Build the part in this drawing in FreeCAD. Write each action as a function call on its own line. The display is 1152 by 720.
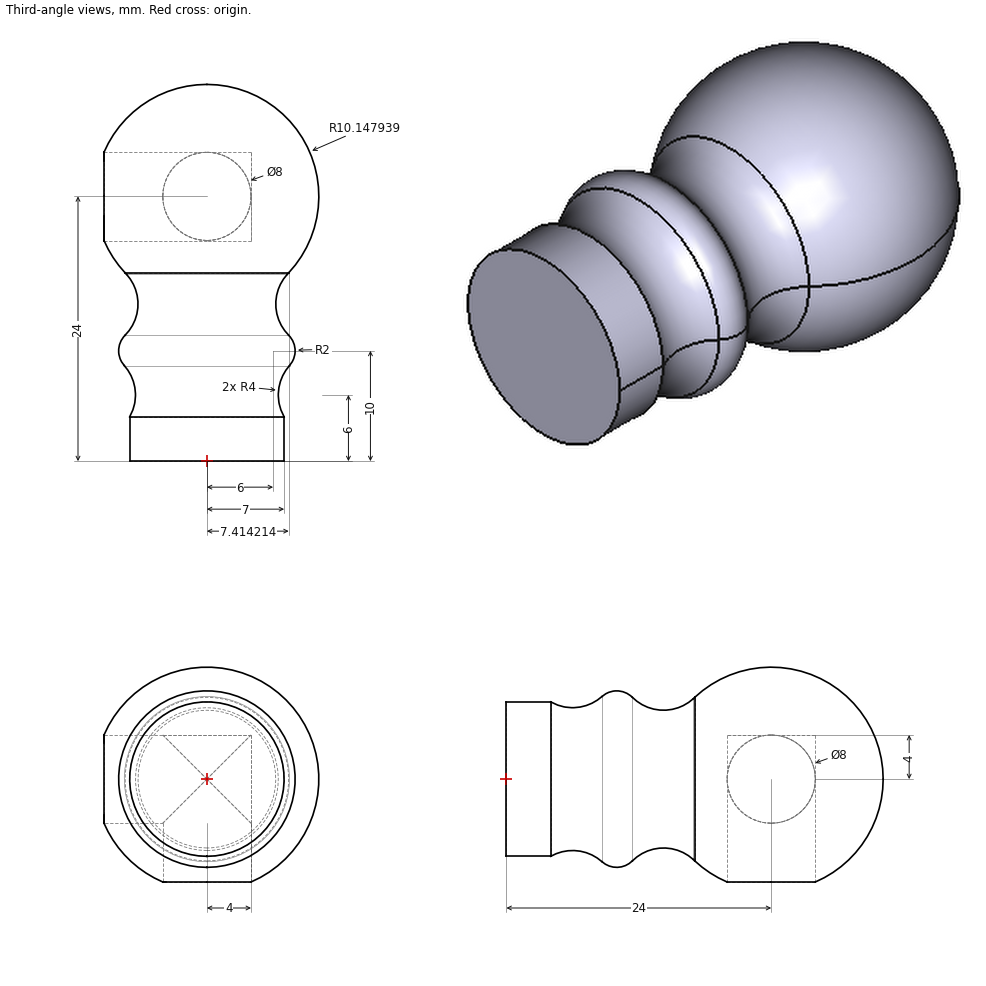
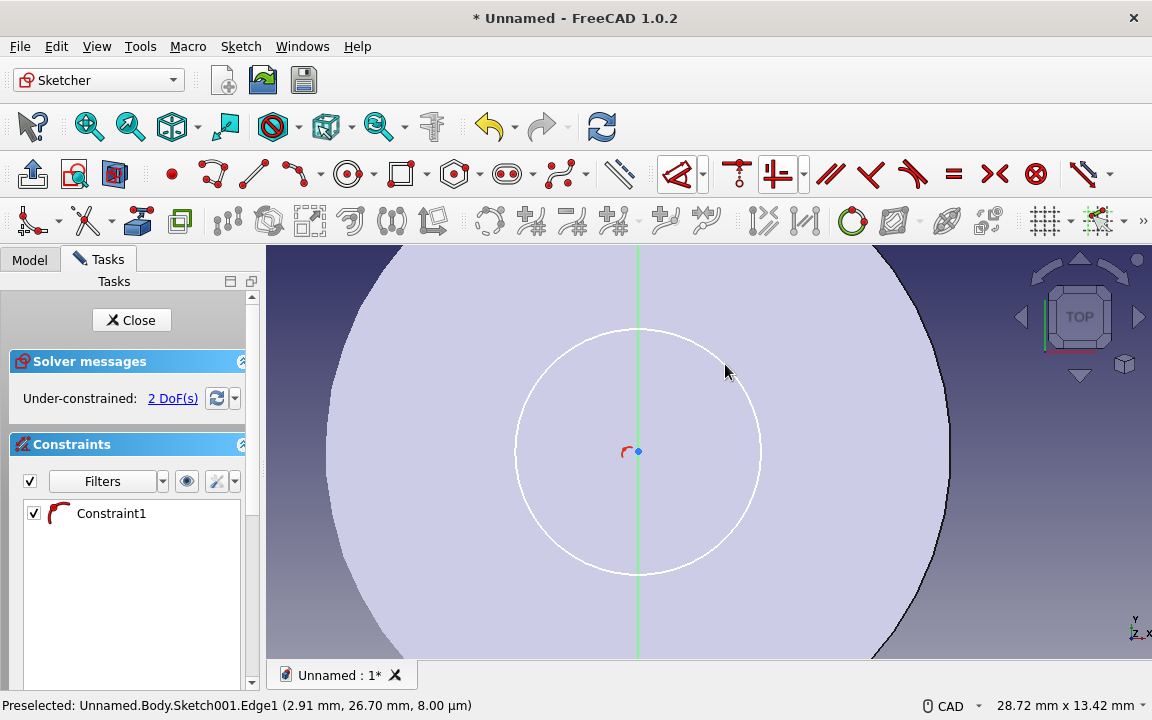
click(725, 365)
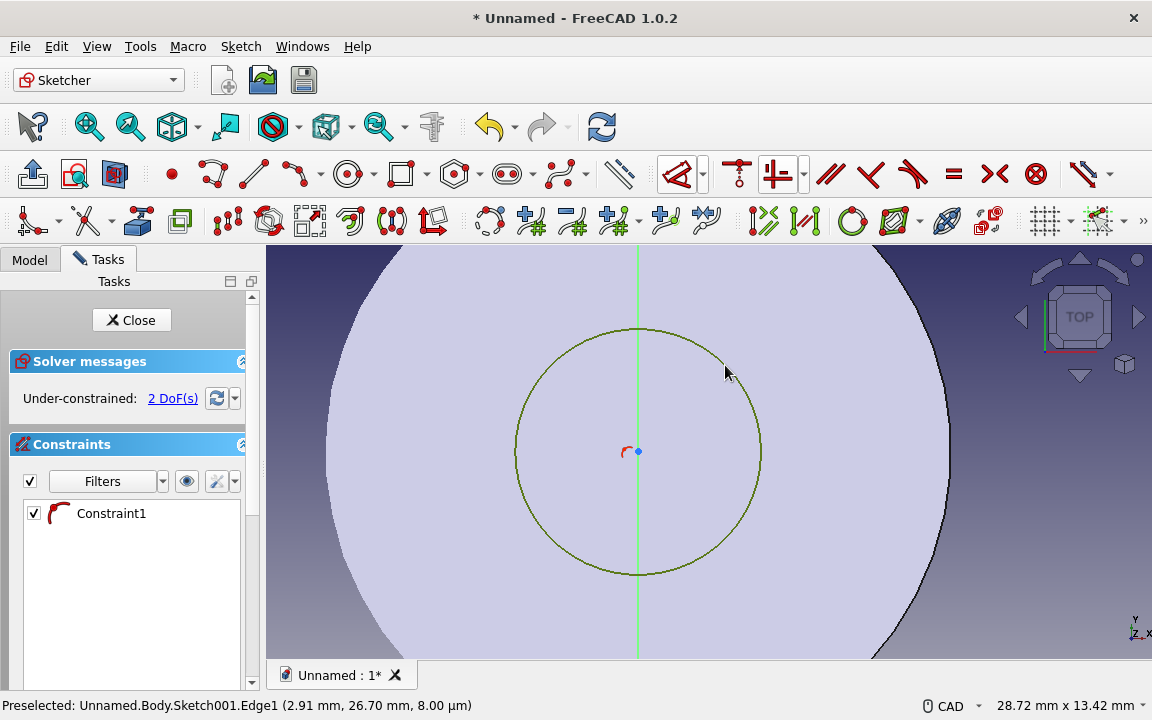
key(k)
key(o)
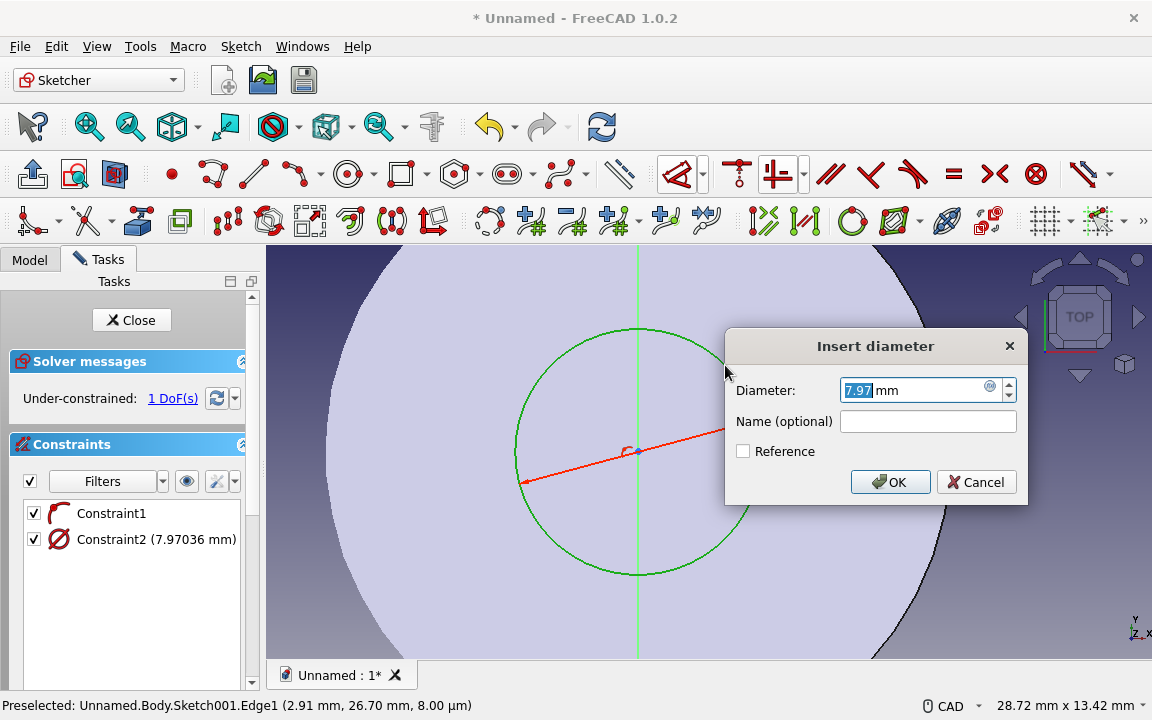
text(8)
key(Return)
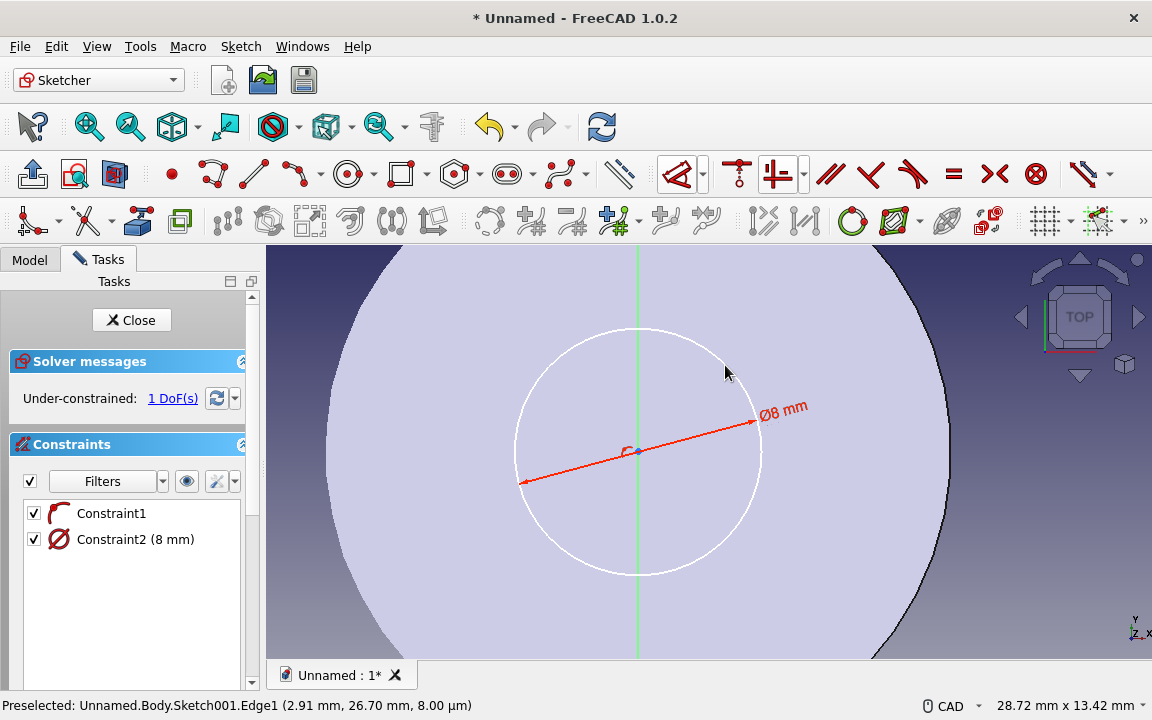
click(638, 452)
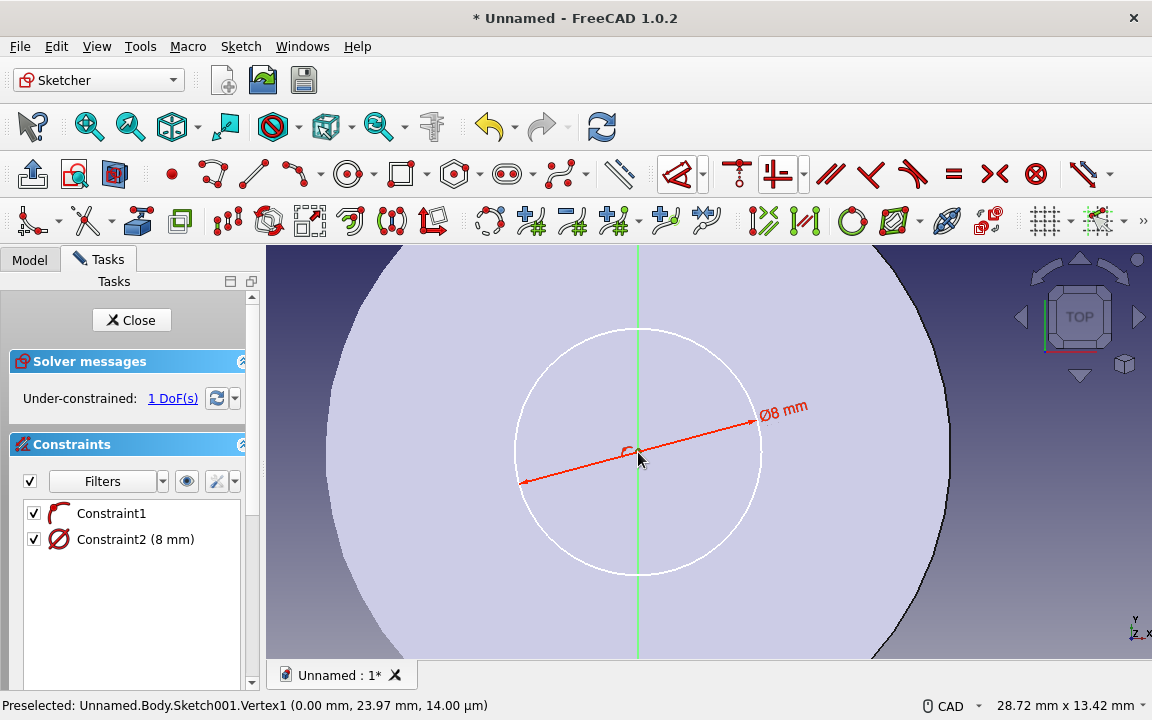
key(i)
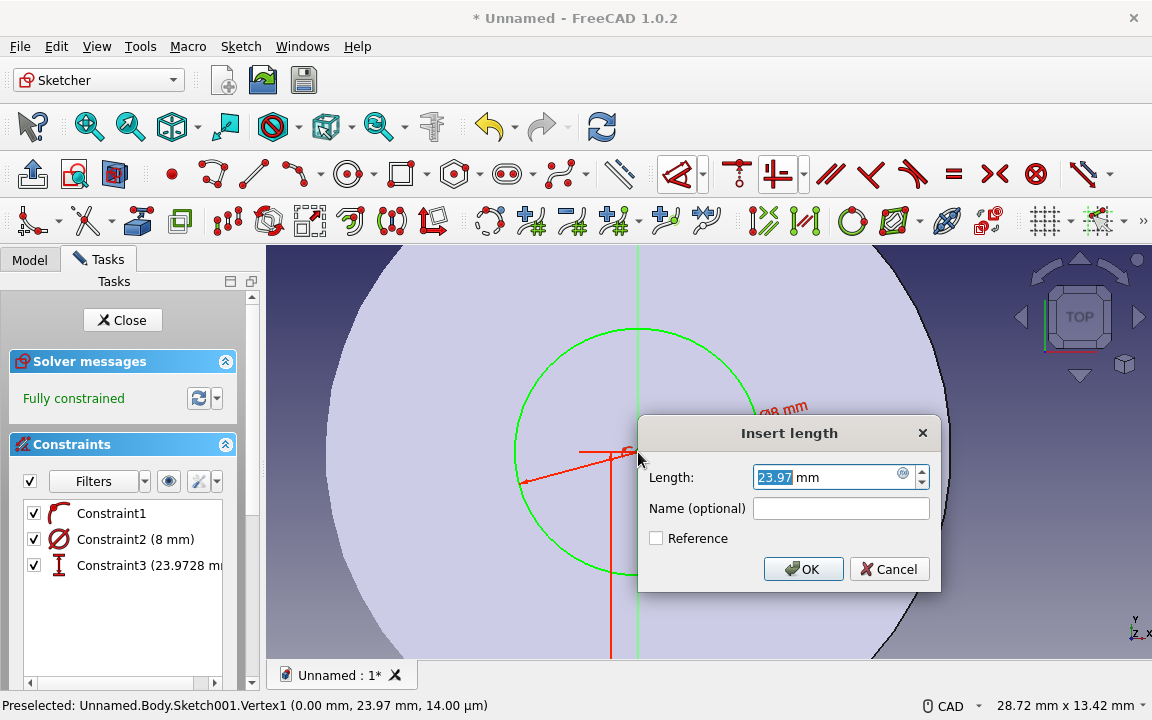
text(24)
key(Return)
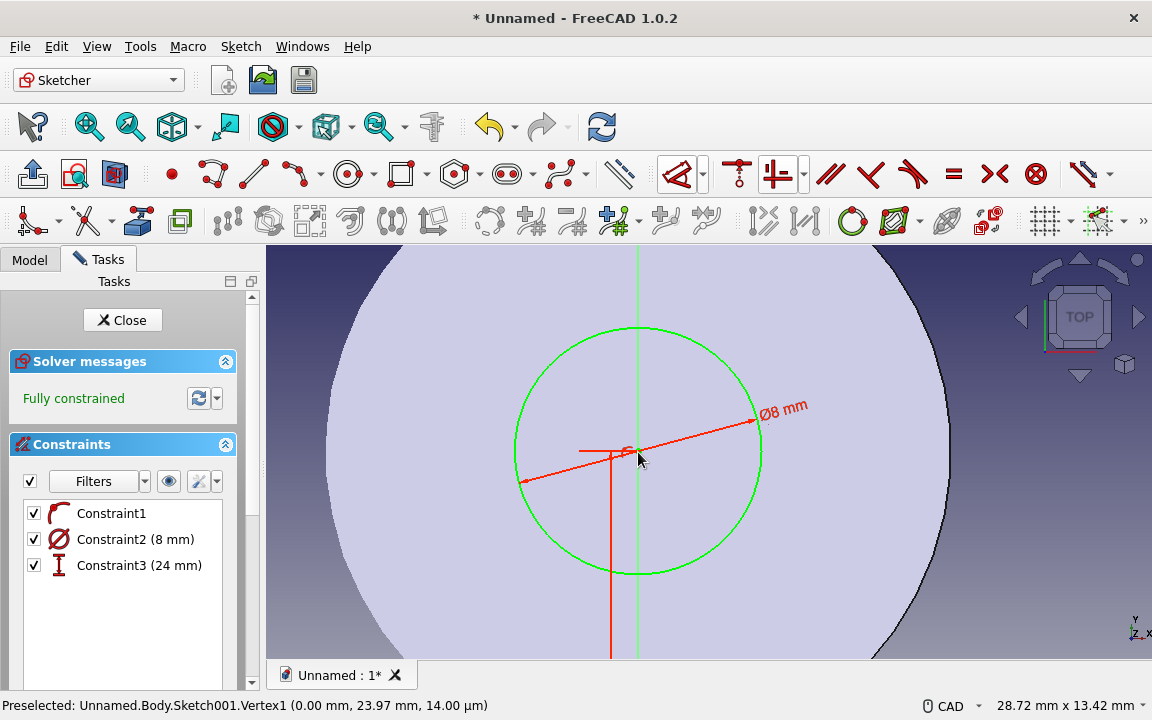
click(123, 320)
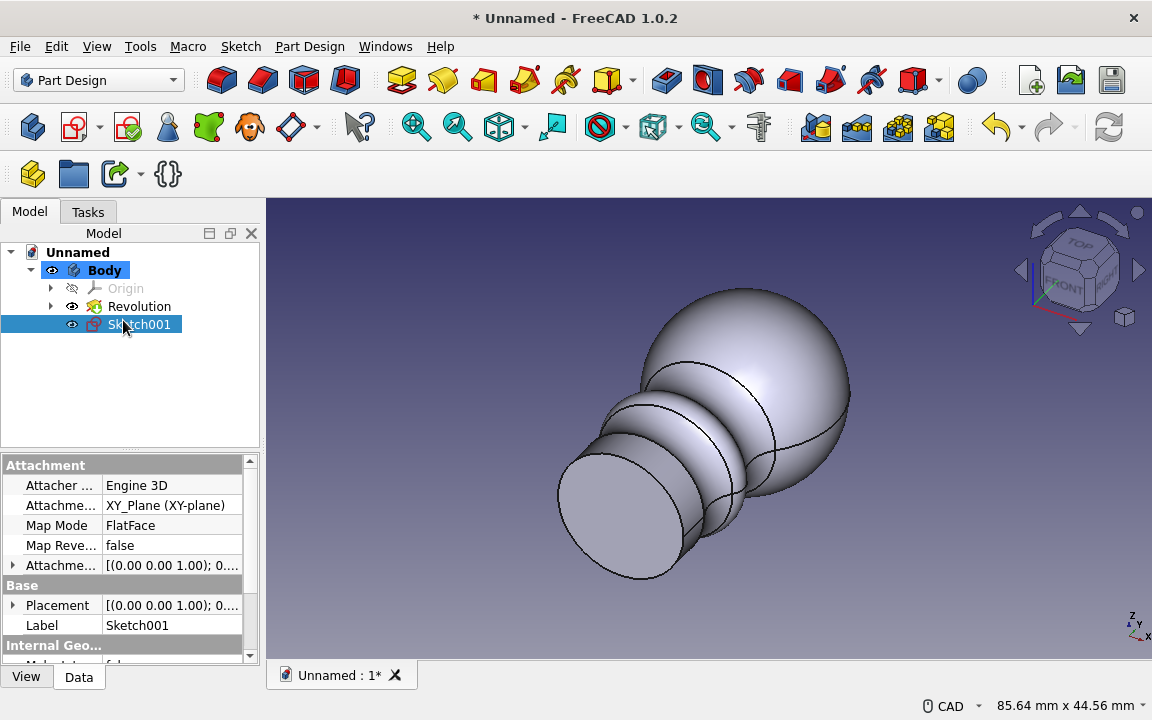
click(667, 80)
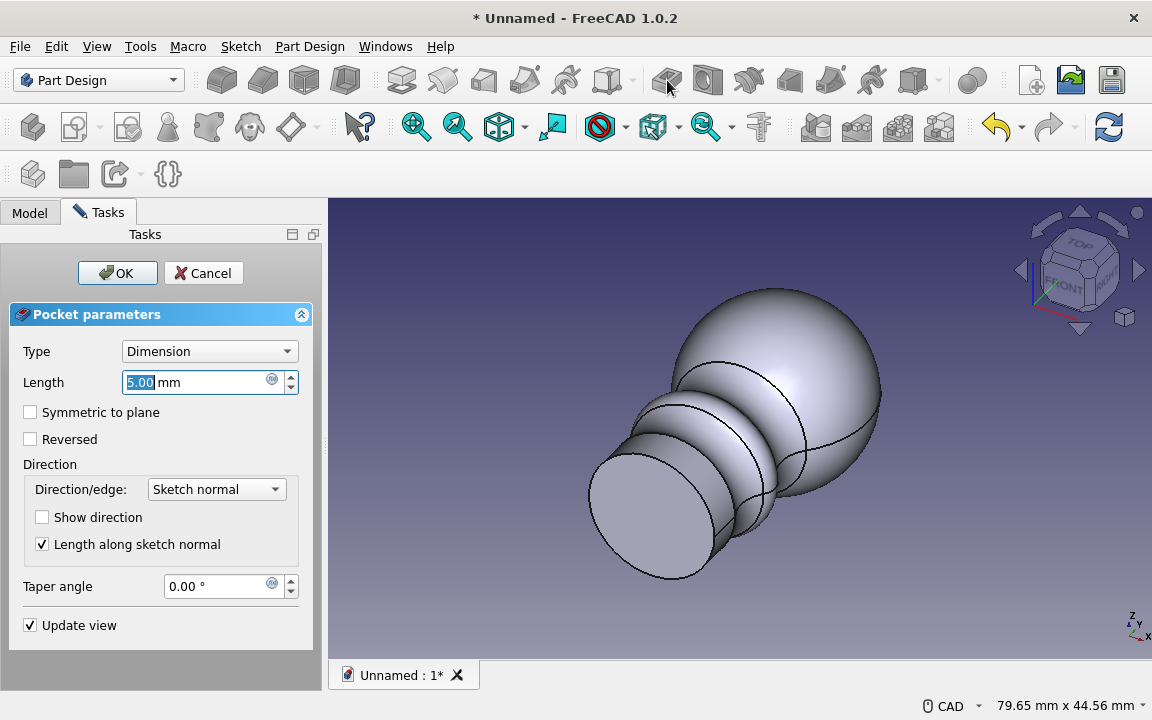
click(210, 352)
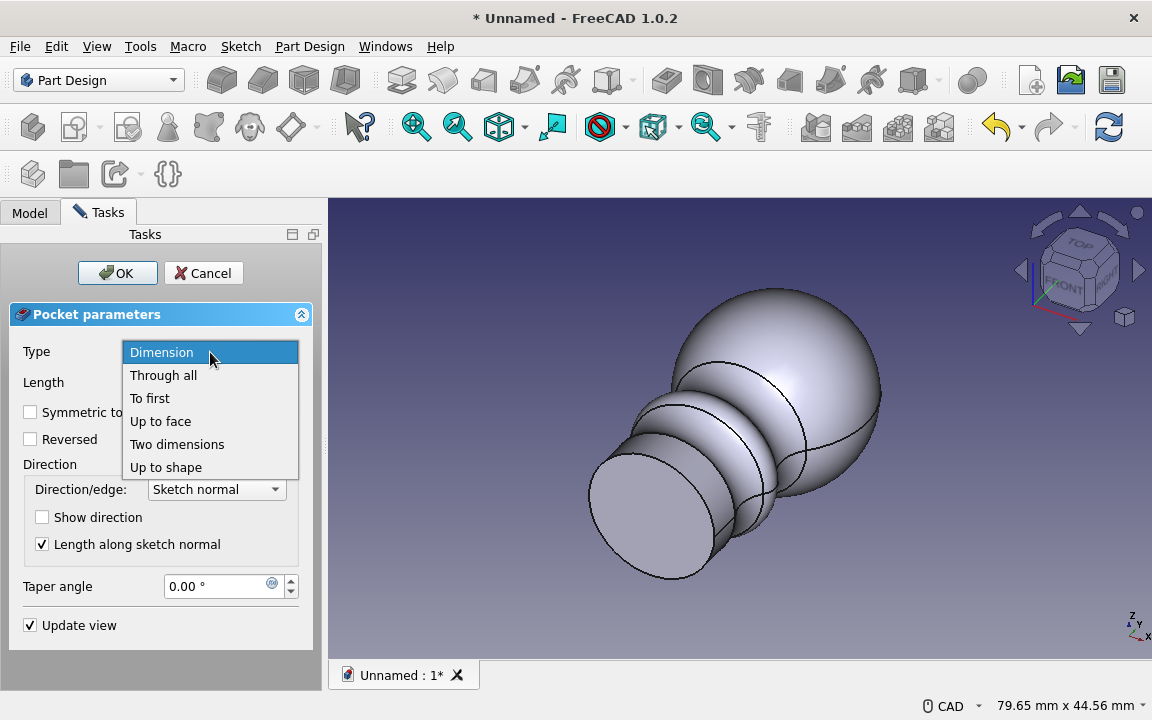
click(208, 444)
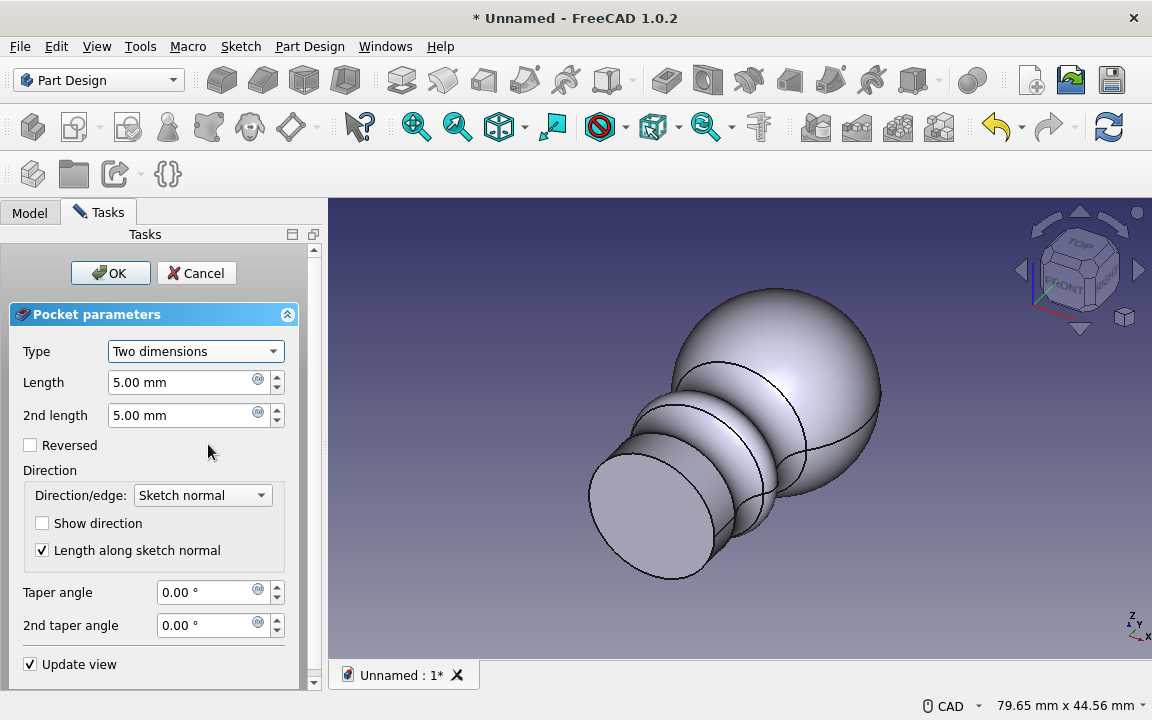
triple_click(190, 382)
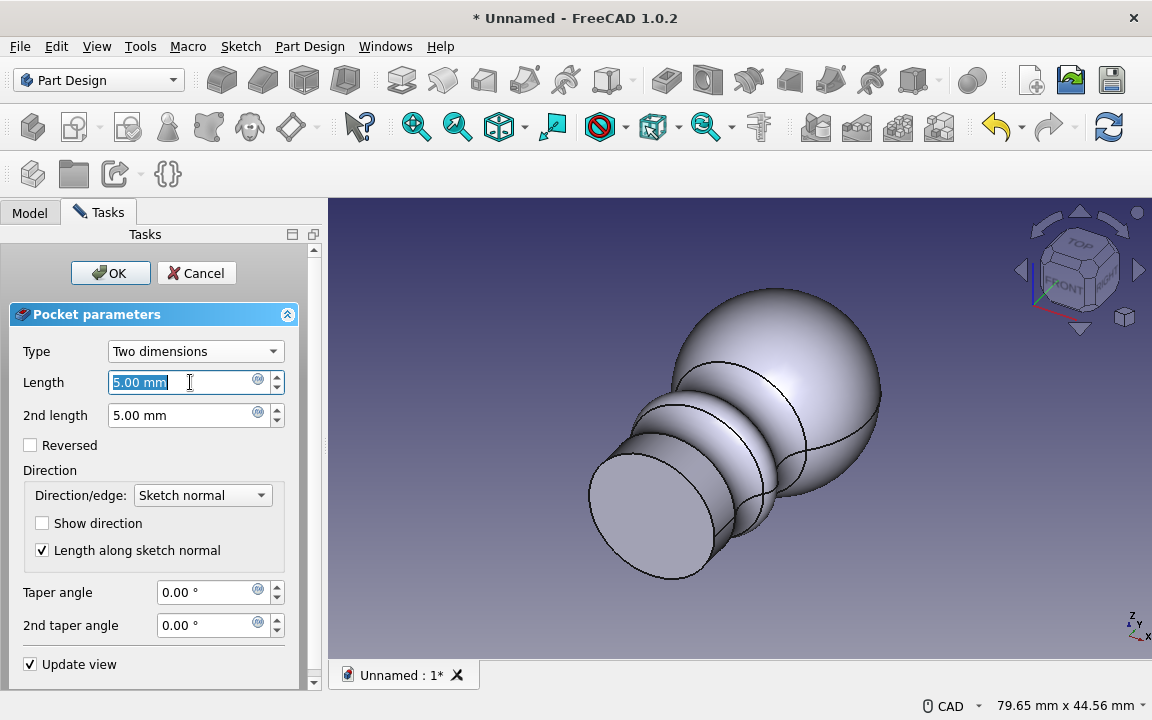
text(4)
key(Tab)